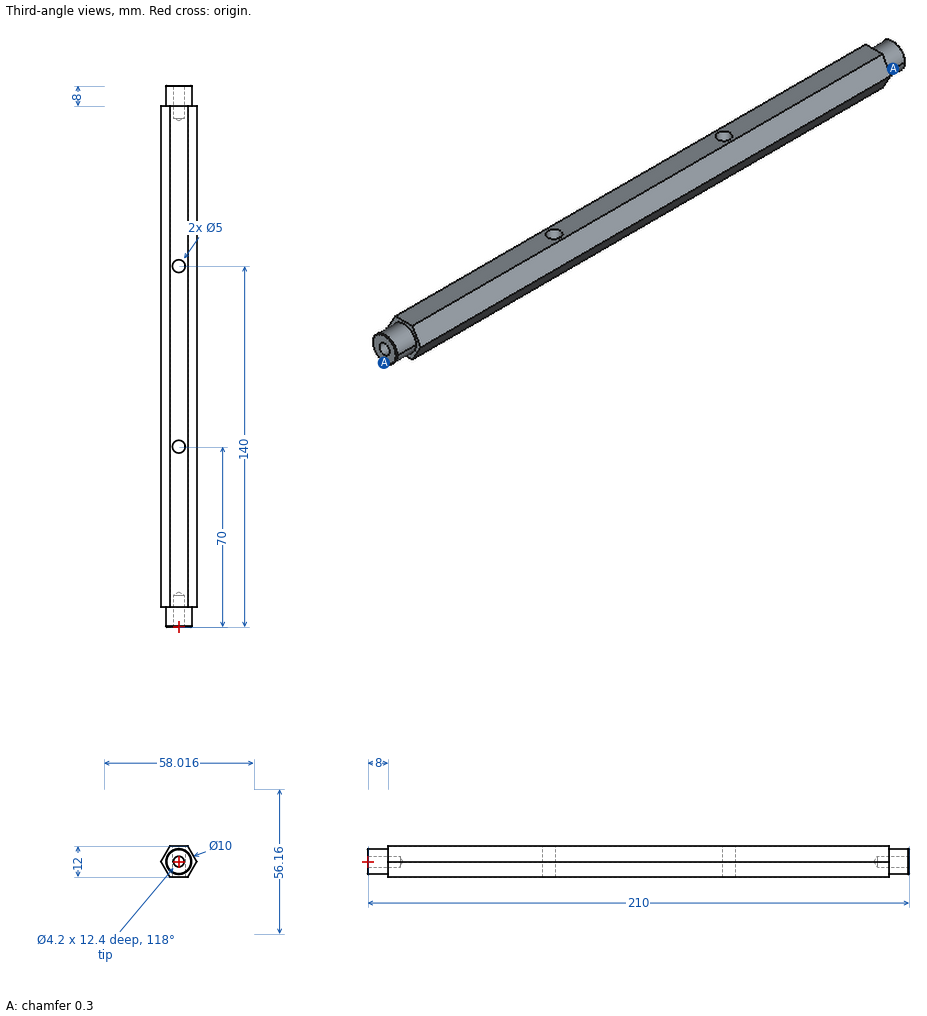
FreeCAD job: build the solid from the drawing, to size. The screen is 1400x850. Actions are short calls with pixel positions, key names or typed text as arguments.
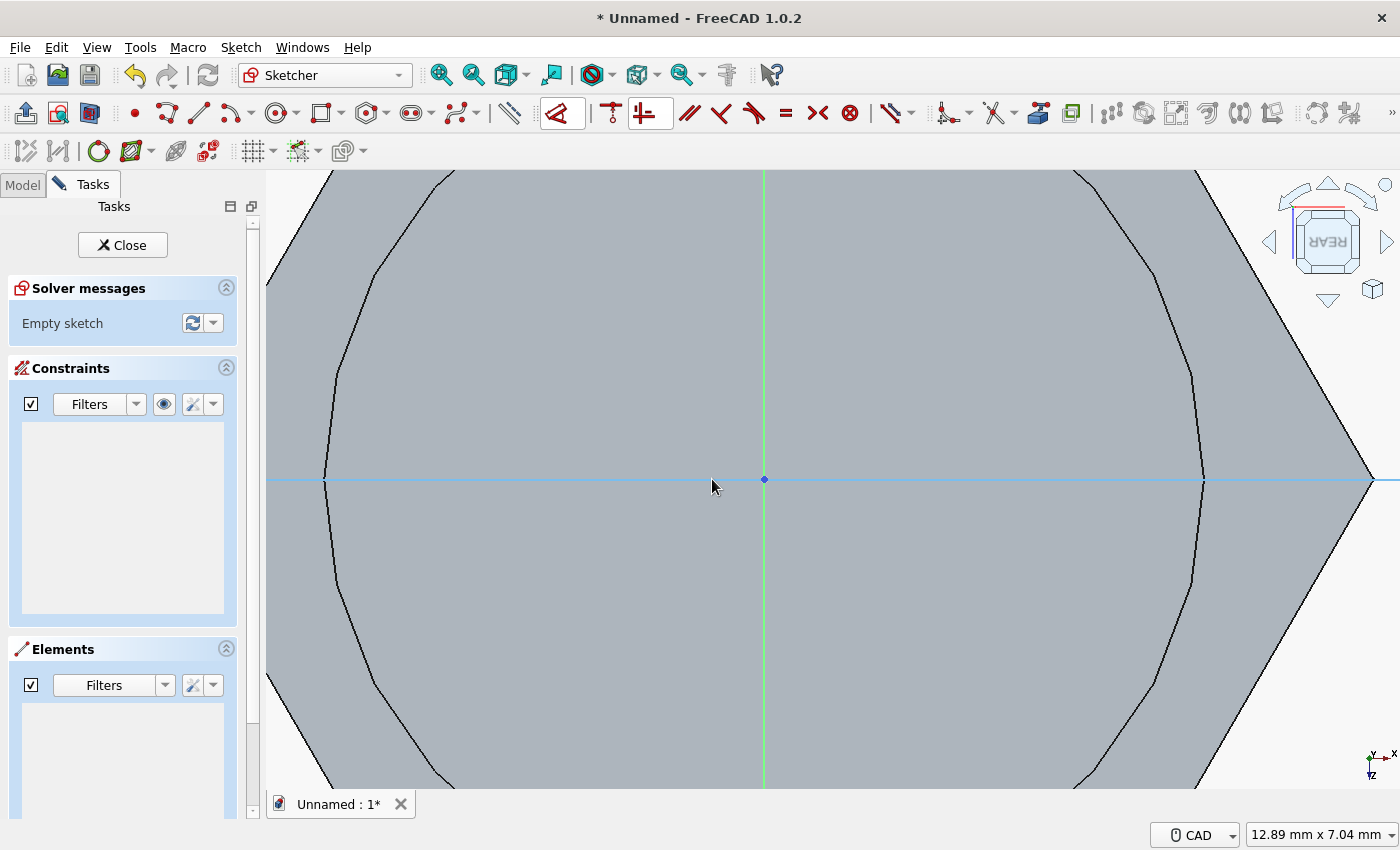
key(g)
key(c)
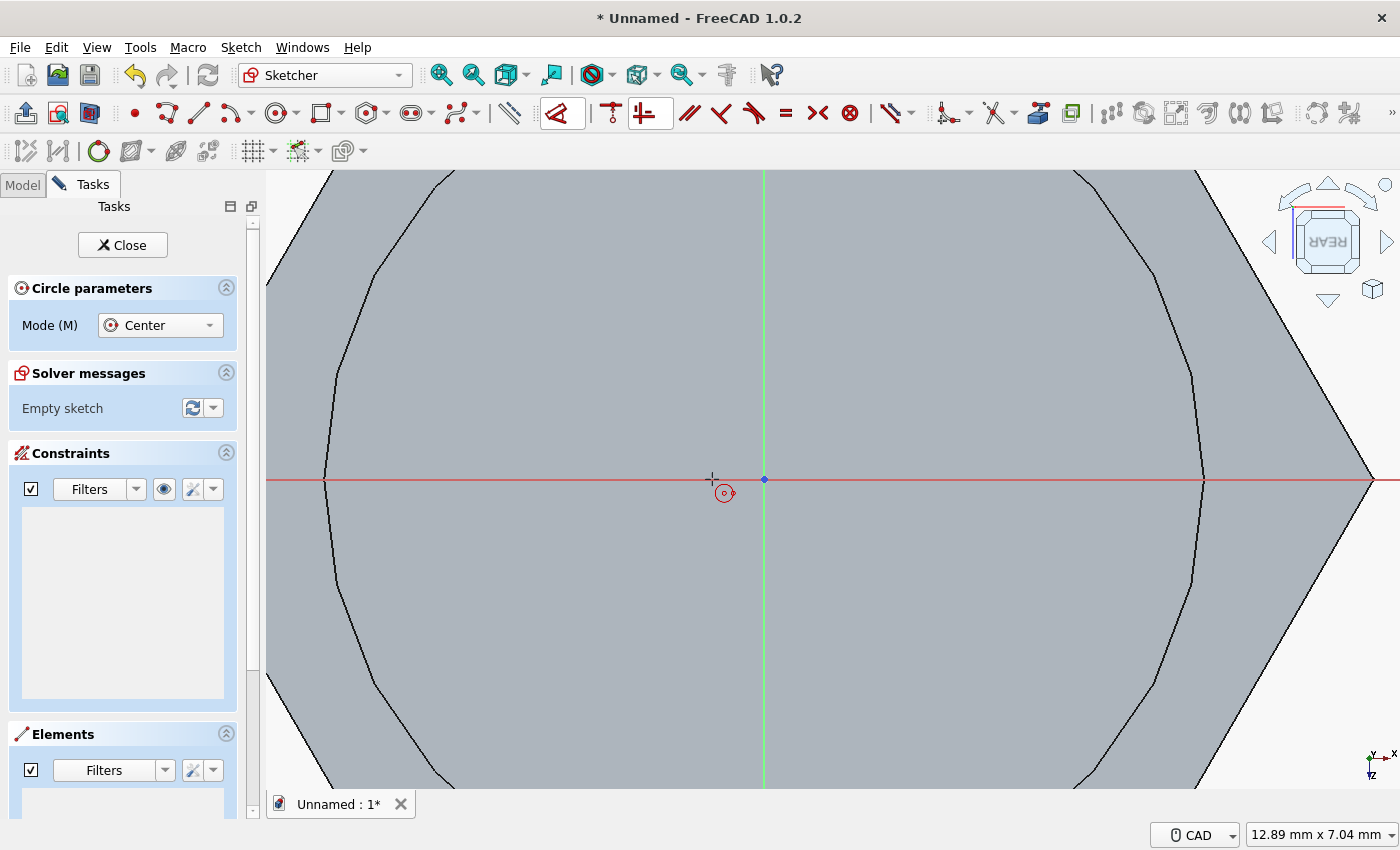
click(764, 479)
click(895, 349)
key(Escape)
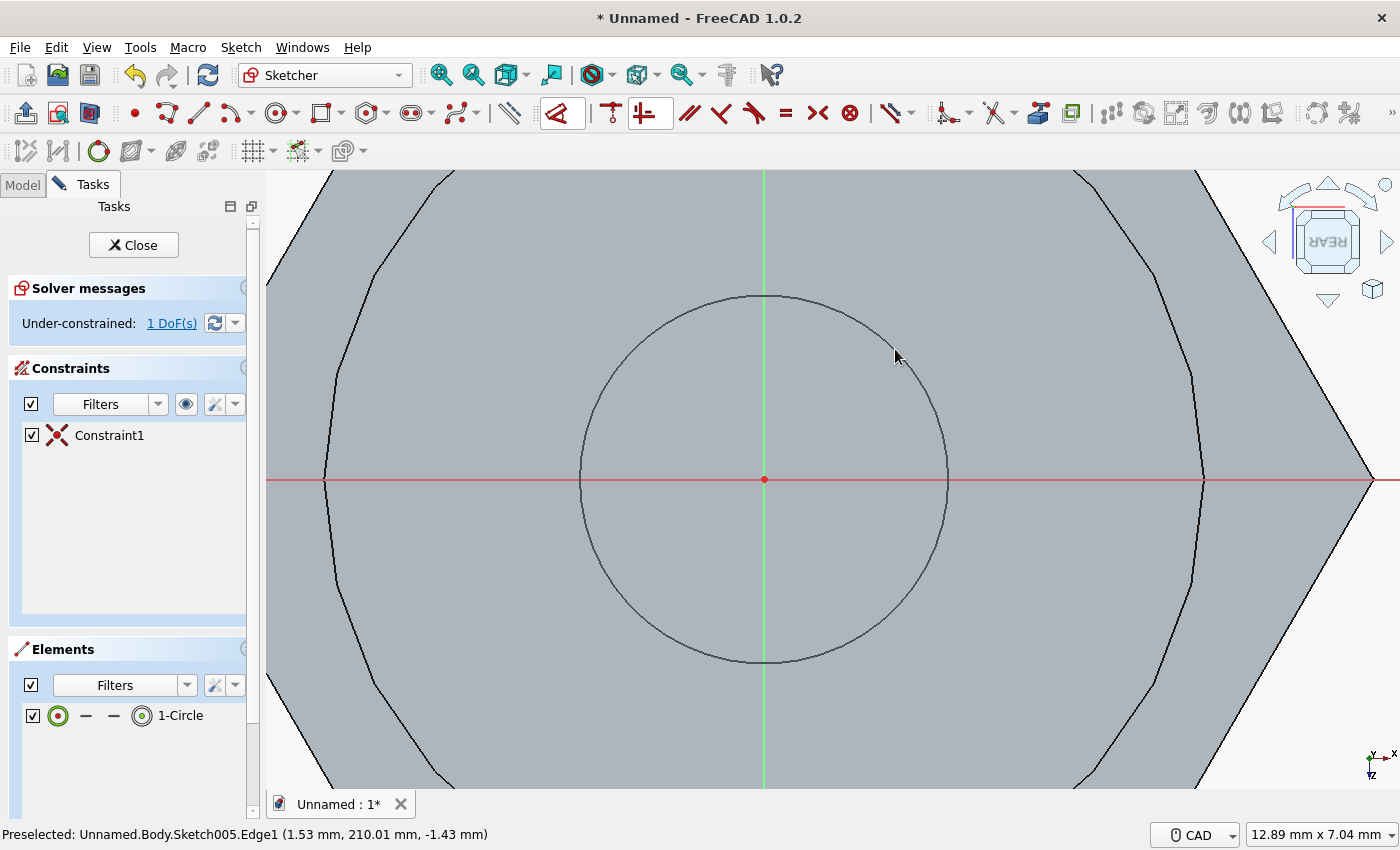
click(894, 349)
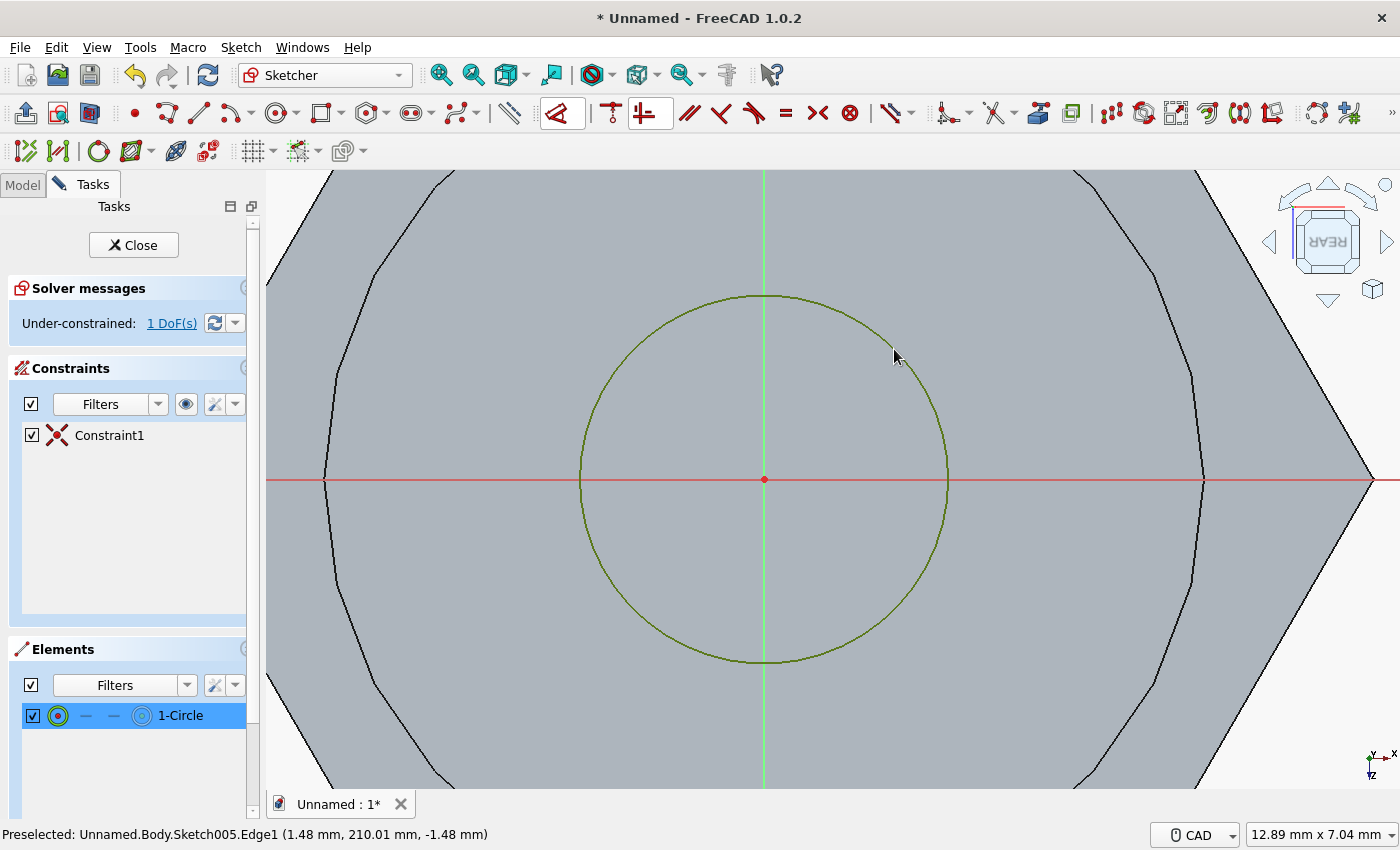
key(k)
key(o)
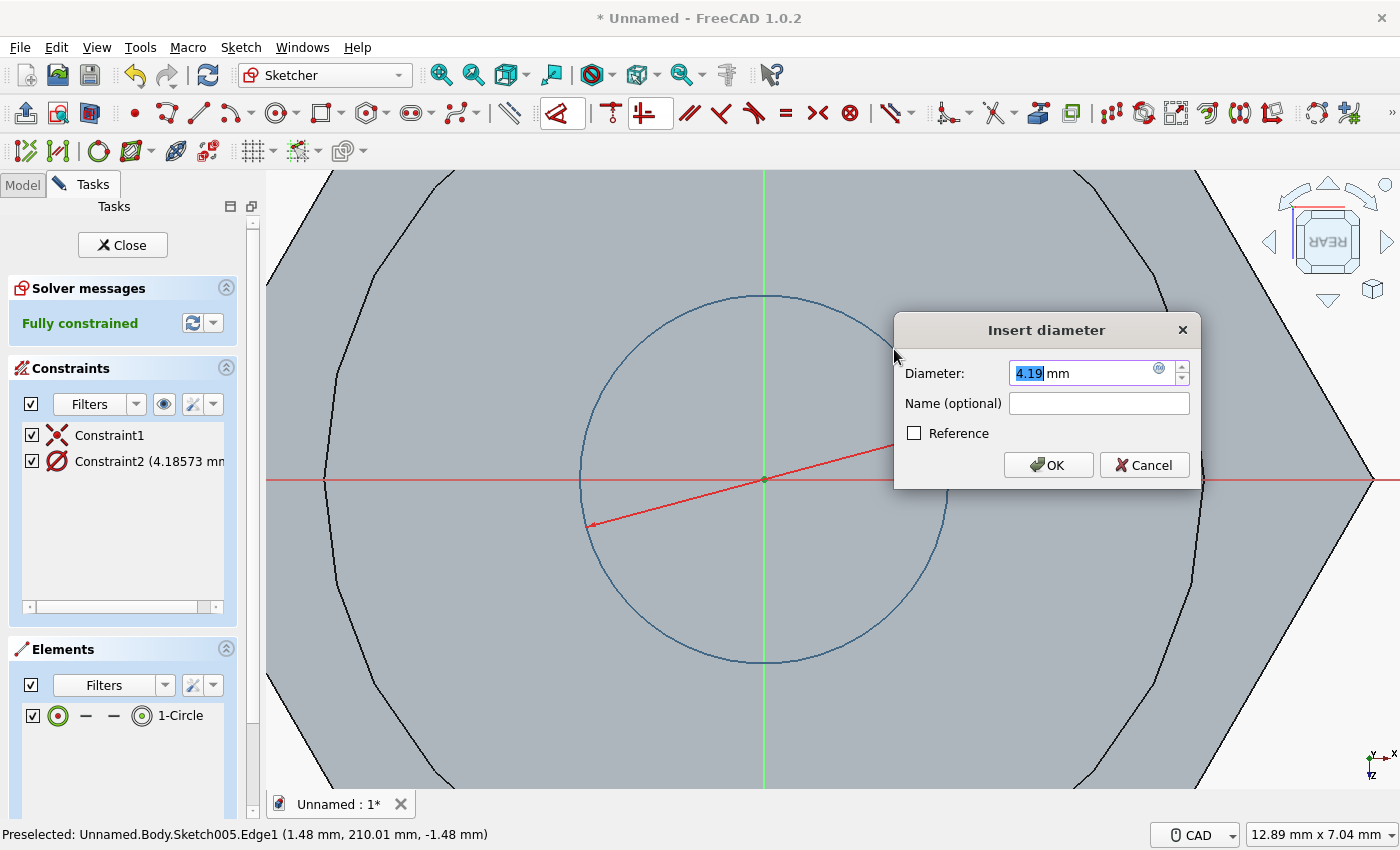
text(4.2)
key(Return)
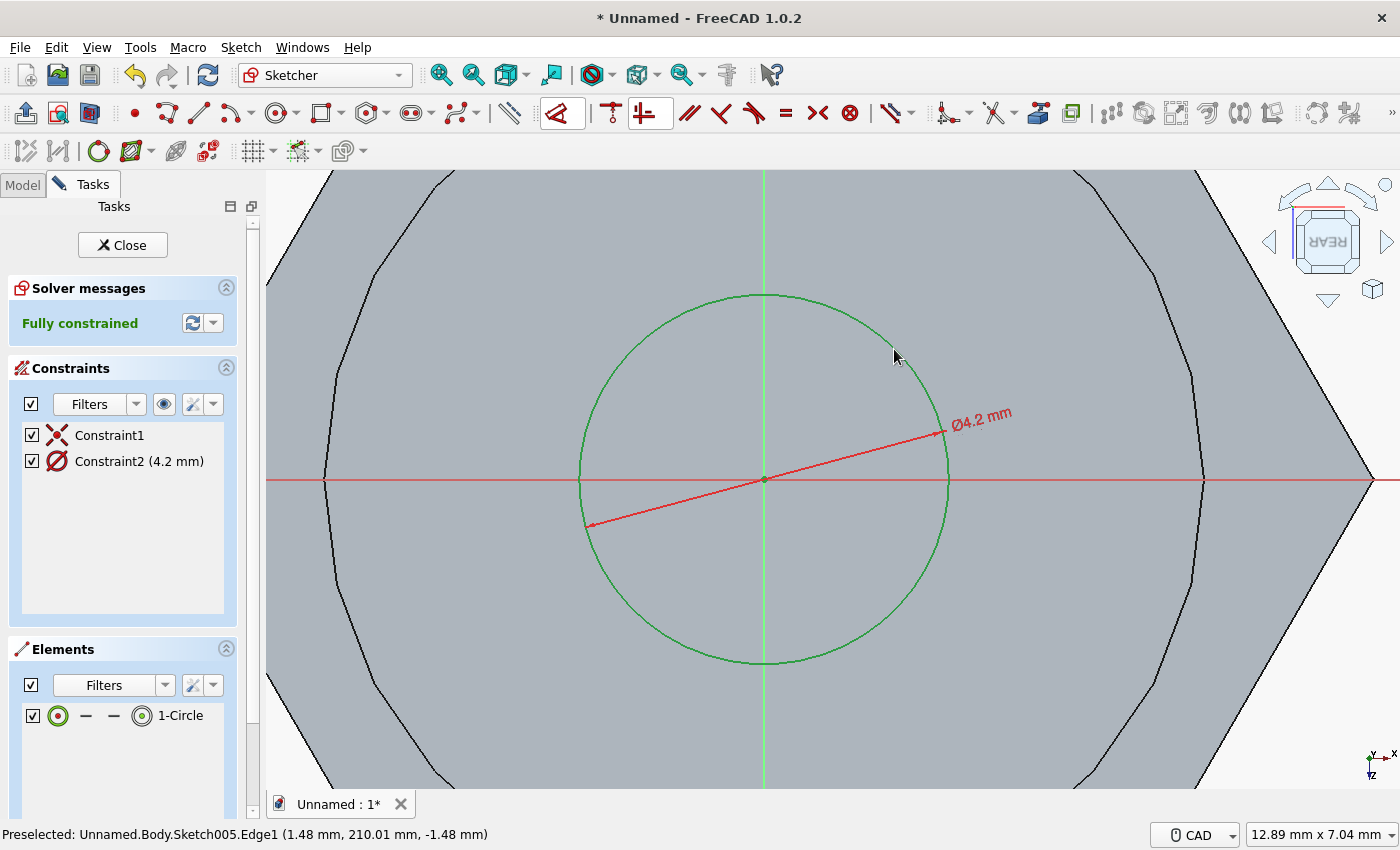
click(123, 245)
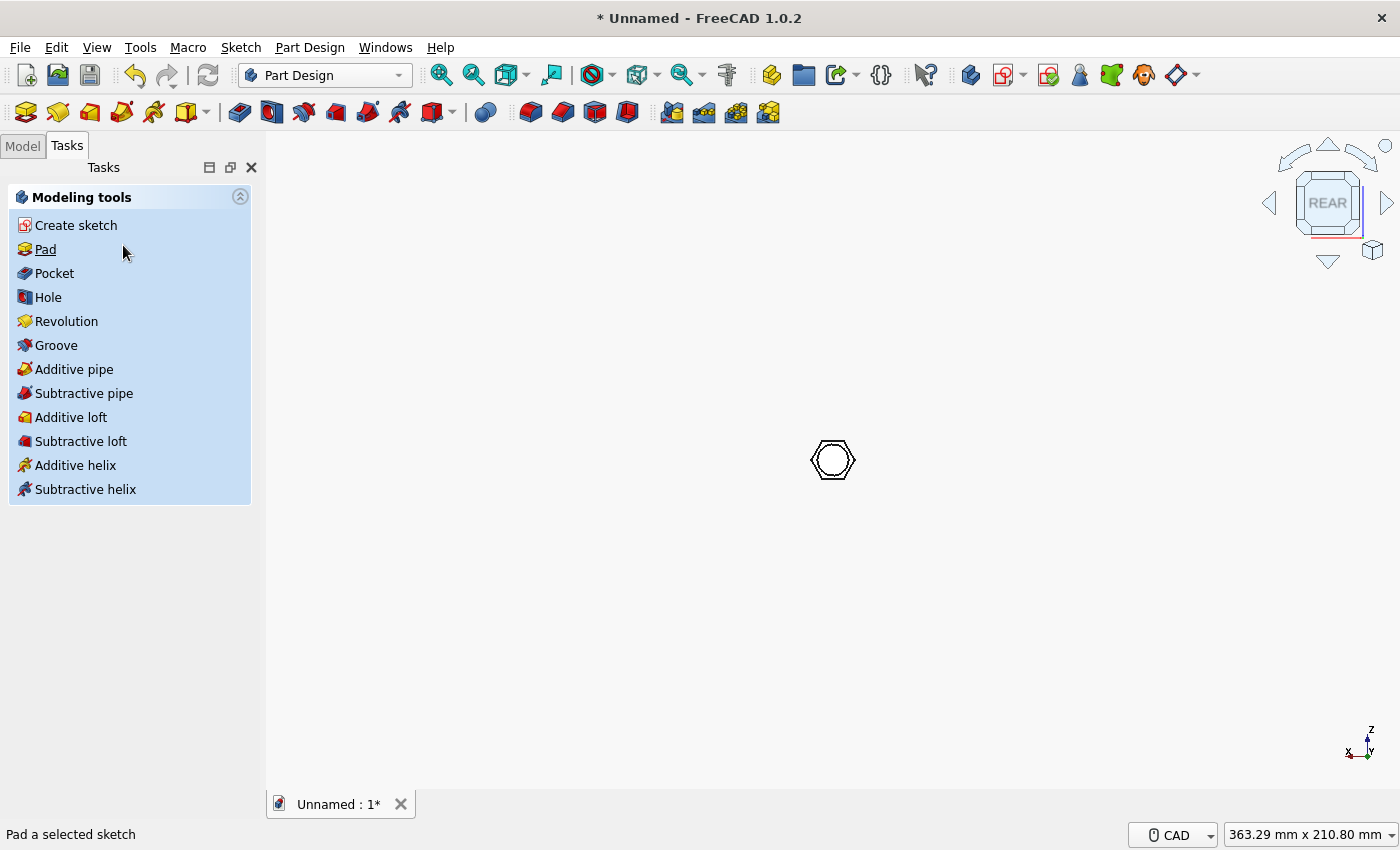
click(272, 112)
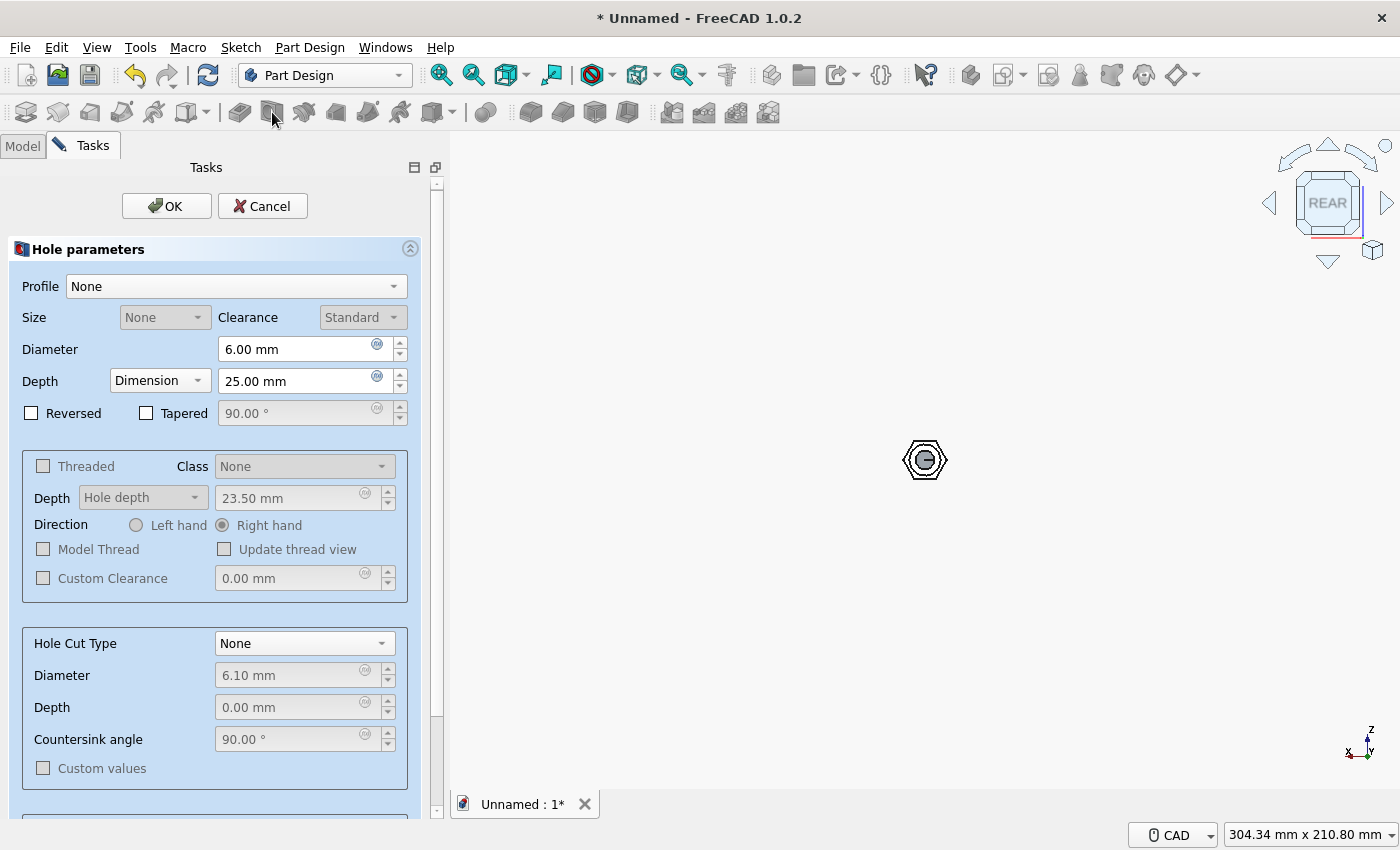
triple_click(305, 349)